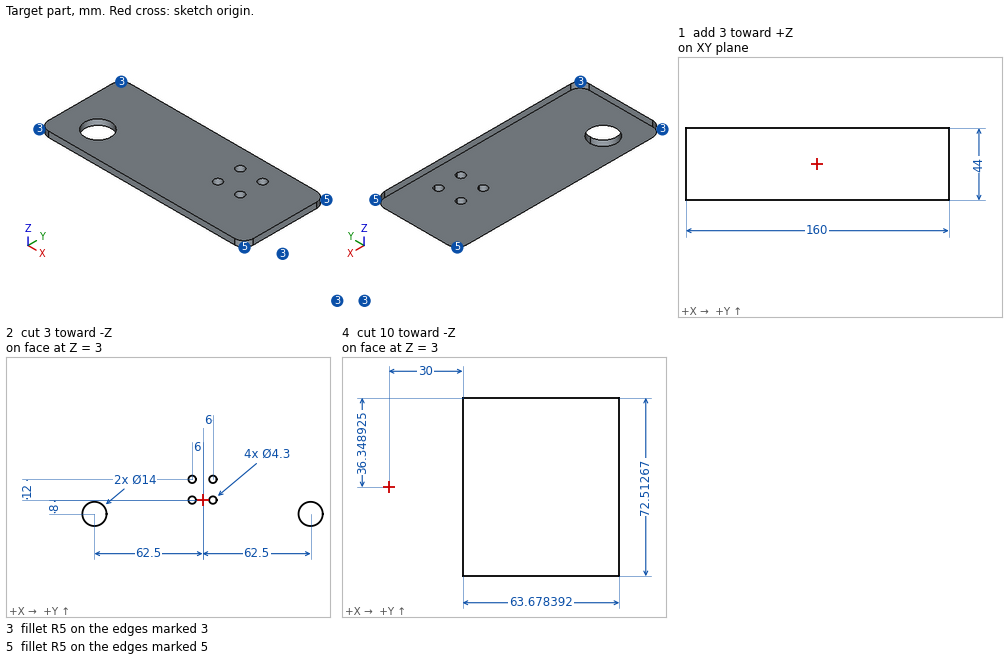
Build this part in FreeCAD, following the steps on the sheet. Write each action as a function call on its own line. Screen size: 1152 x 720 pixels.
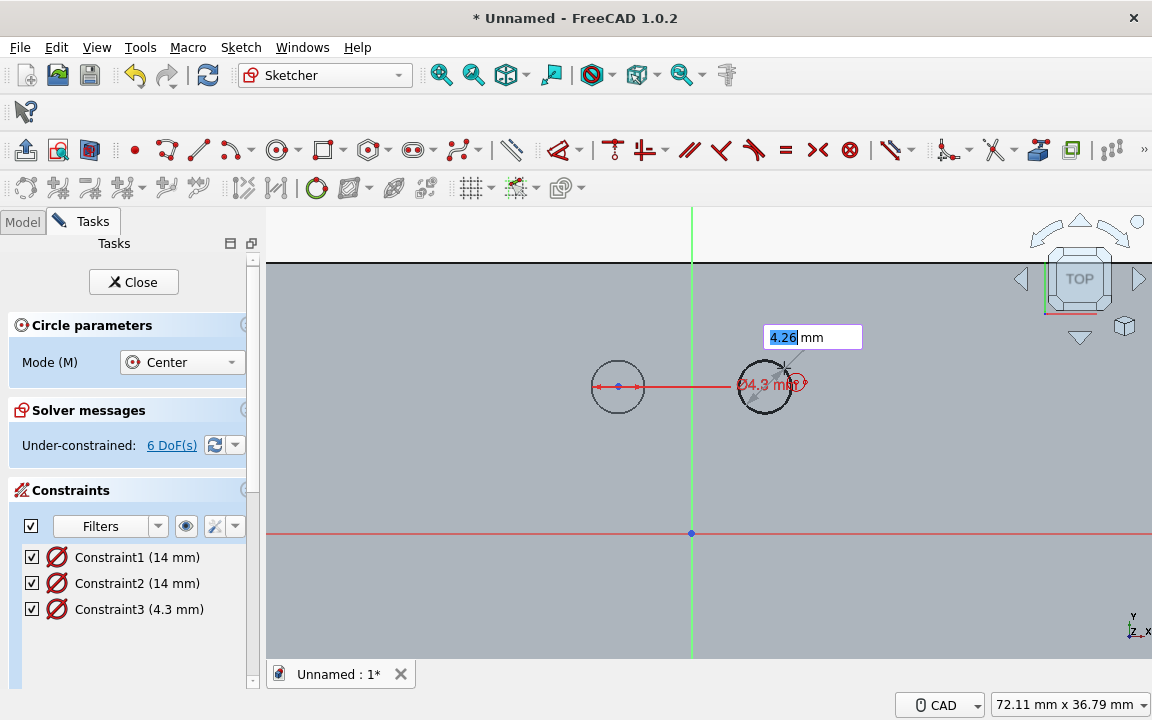
text(4.3)
key(Return)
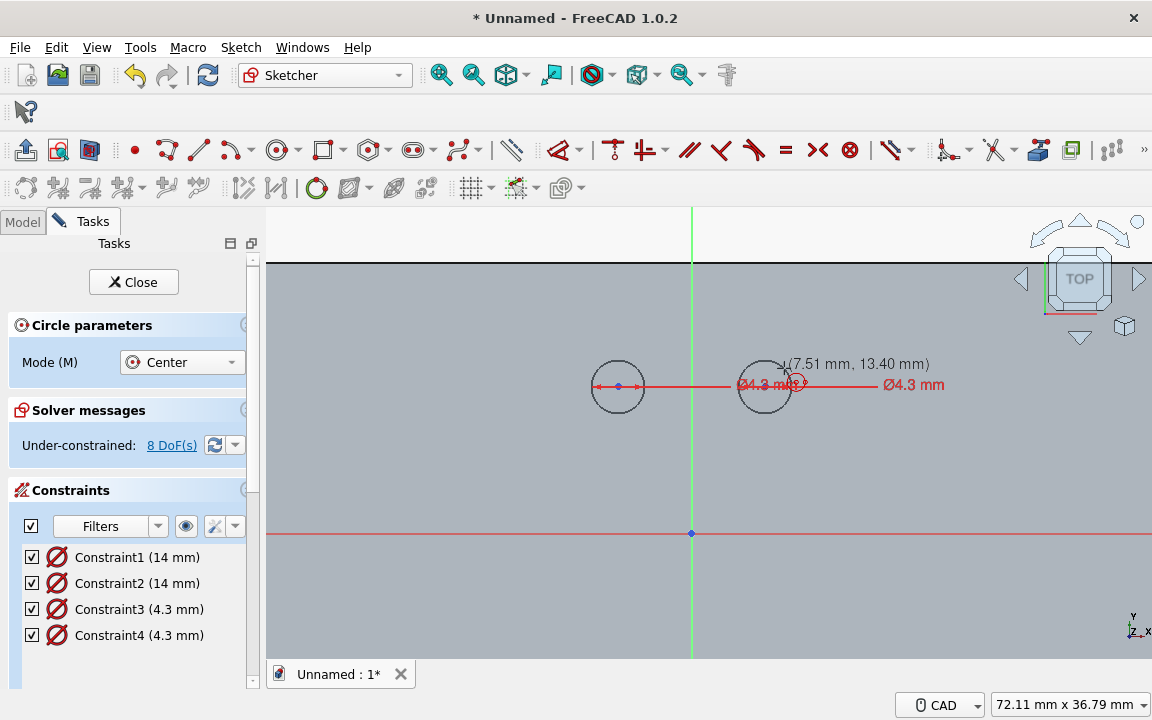
click(765, 534)
move(784, 515)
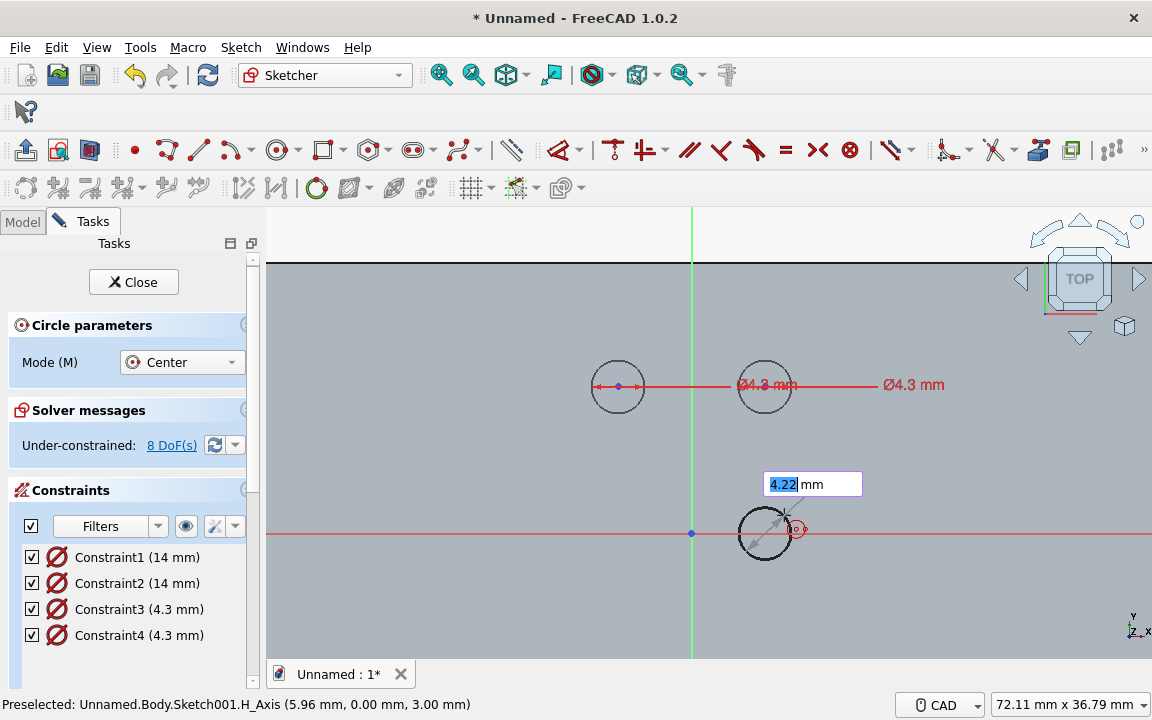
text(4.3)
key(Return)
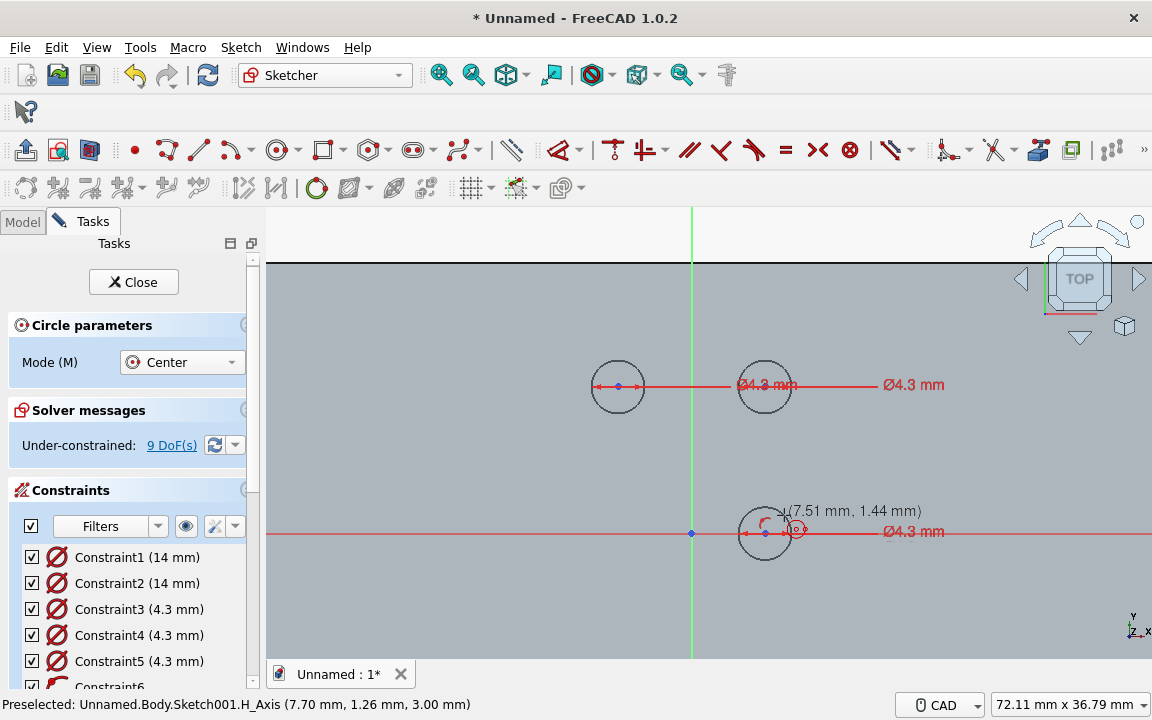
click(618, 534)
move(637, 515)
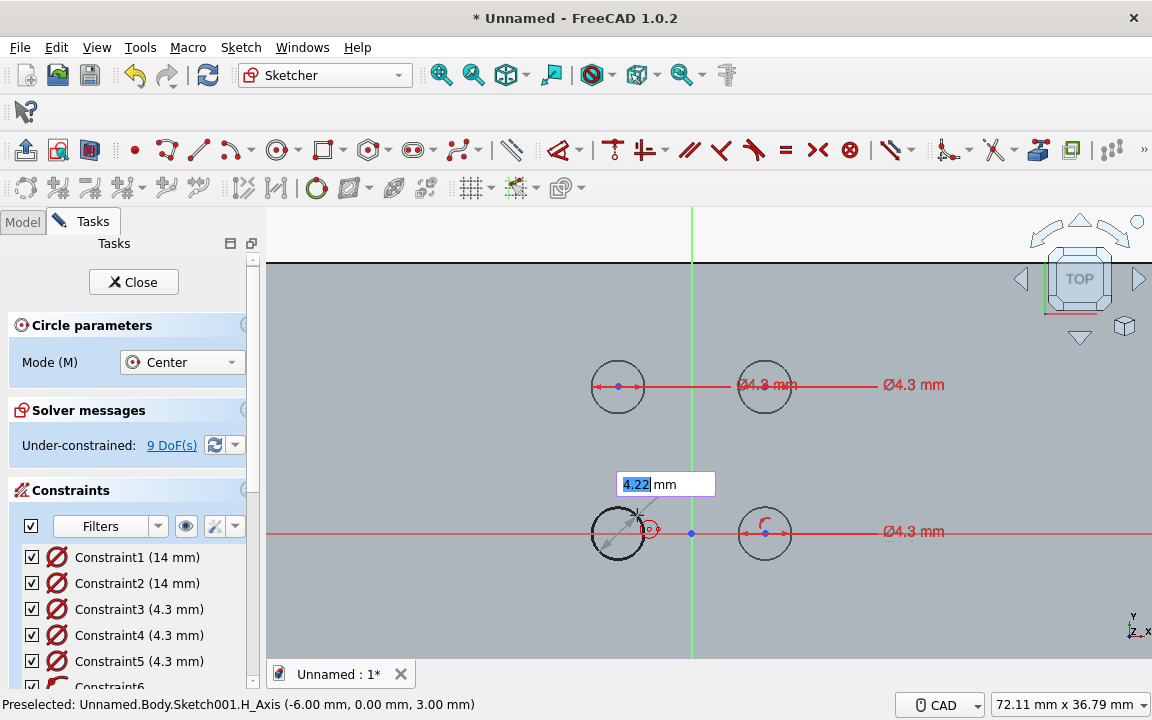
text(4.3)
key(Return)
key(Escape)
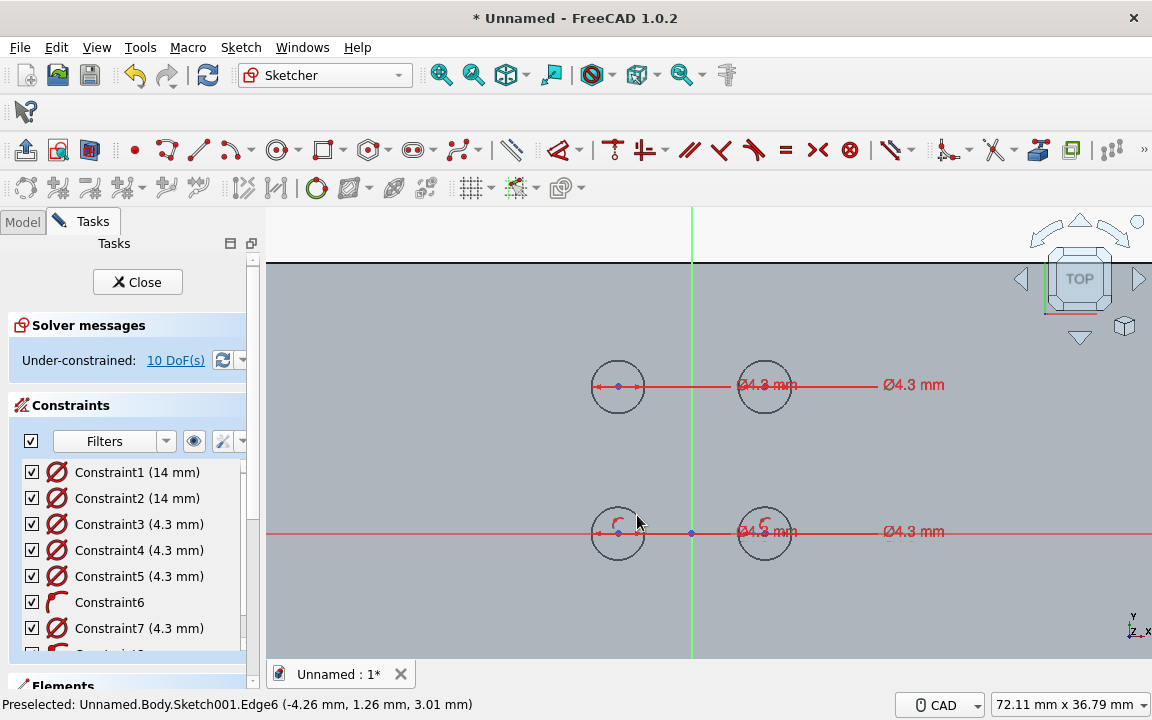
scroll(618, 387, down, 6)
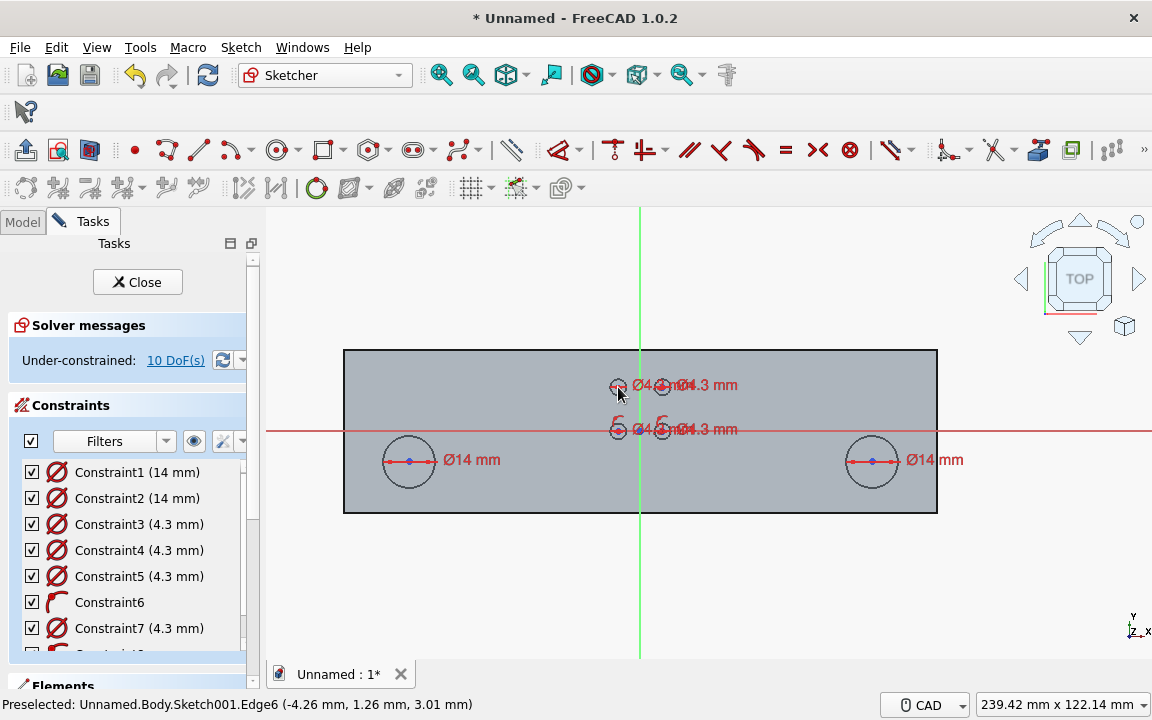
click(409, 462)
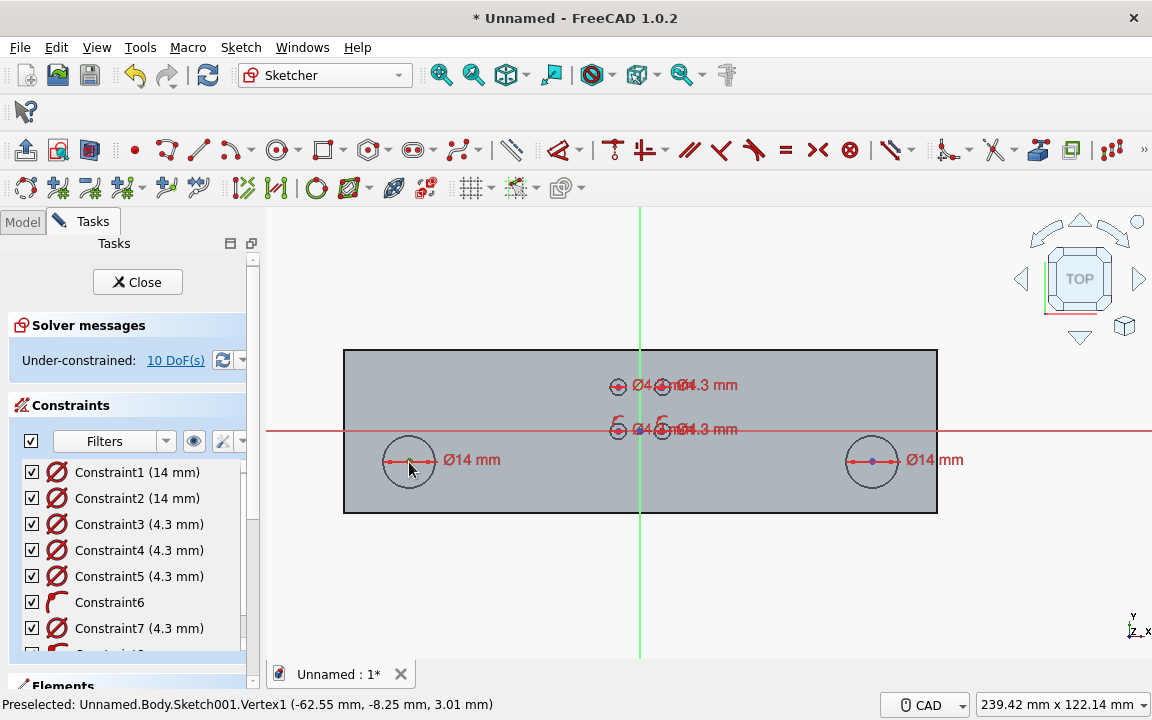
click(872, 462)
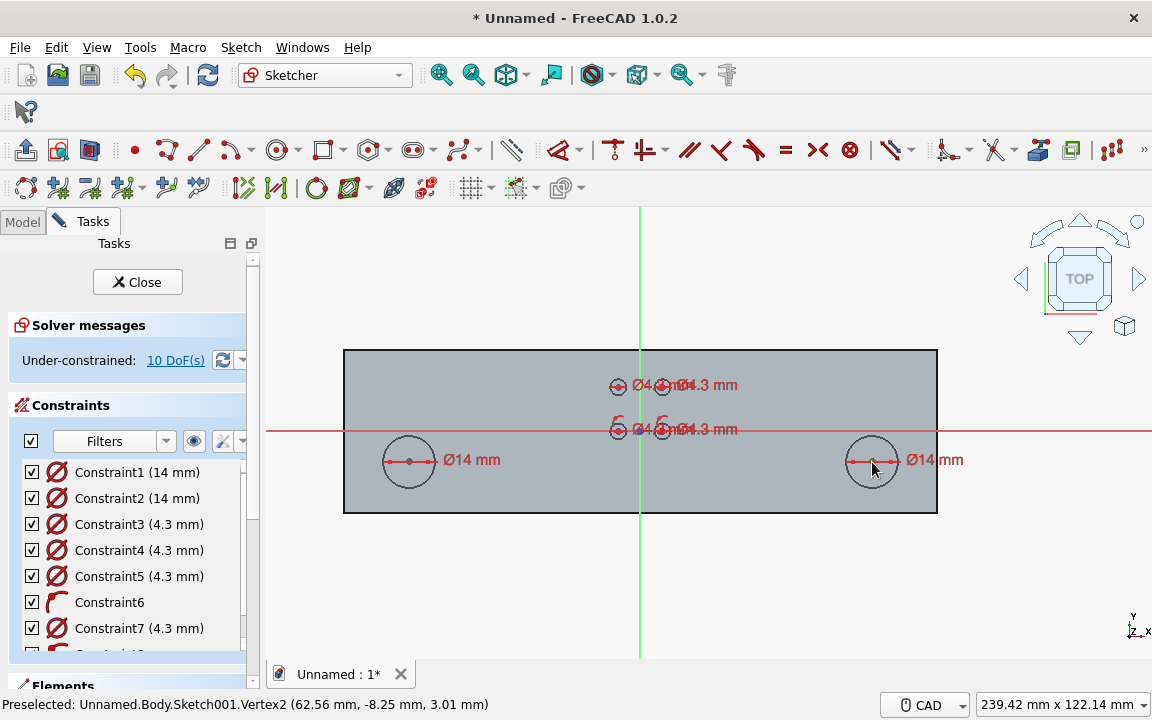
click(668, 150)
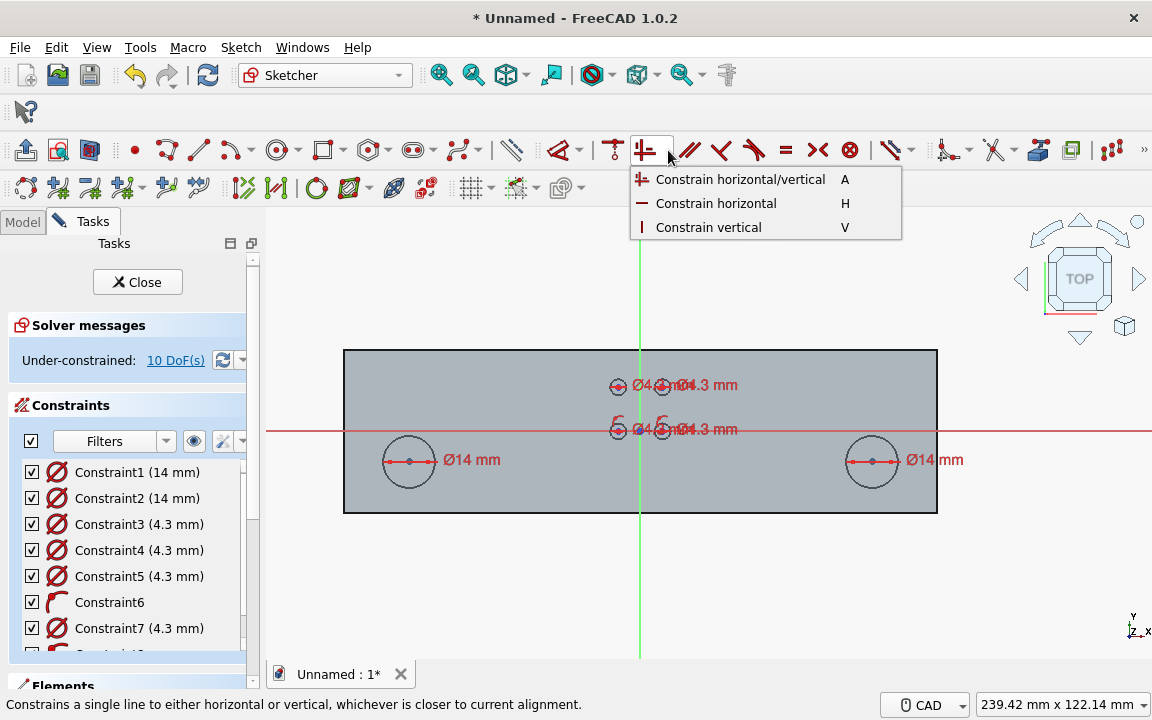
click(766, 203)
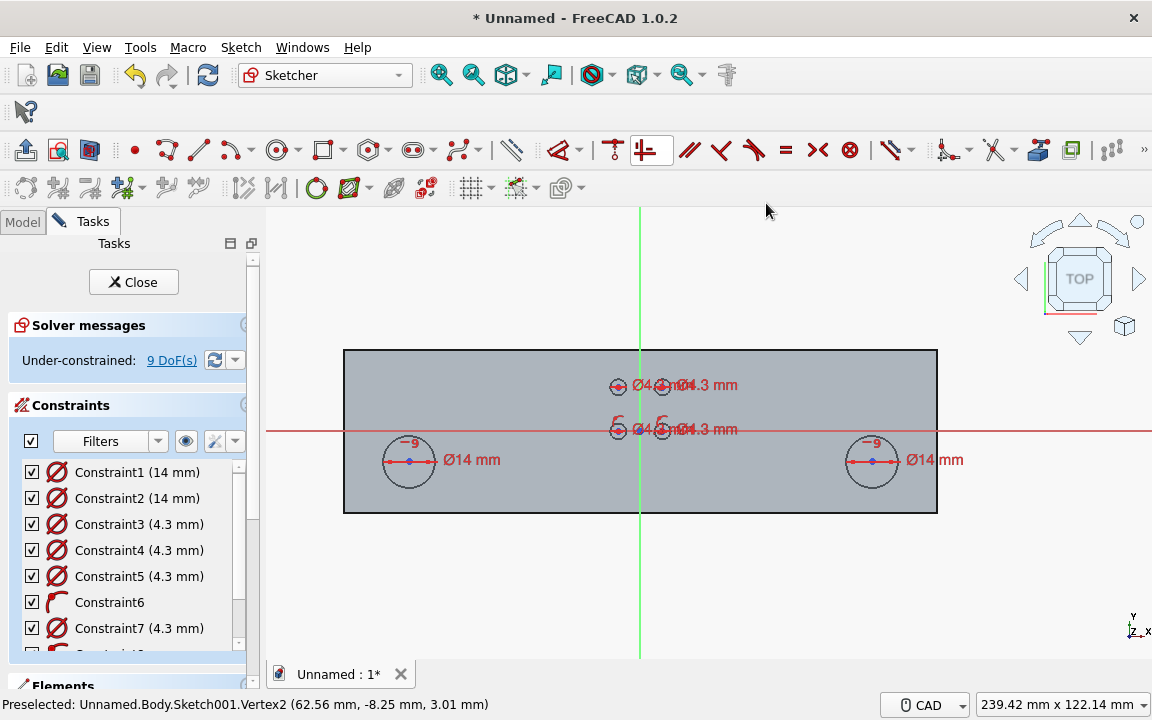
click(618, 387)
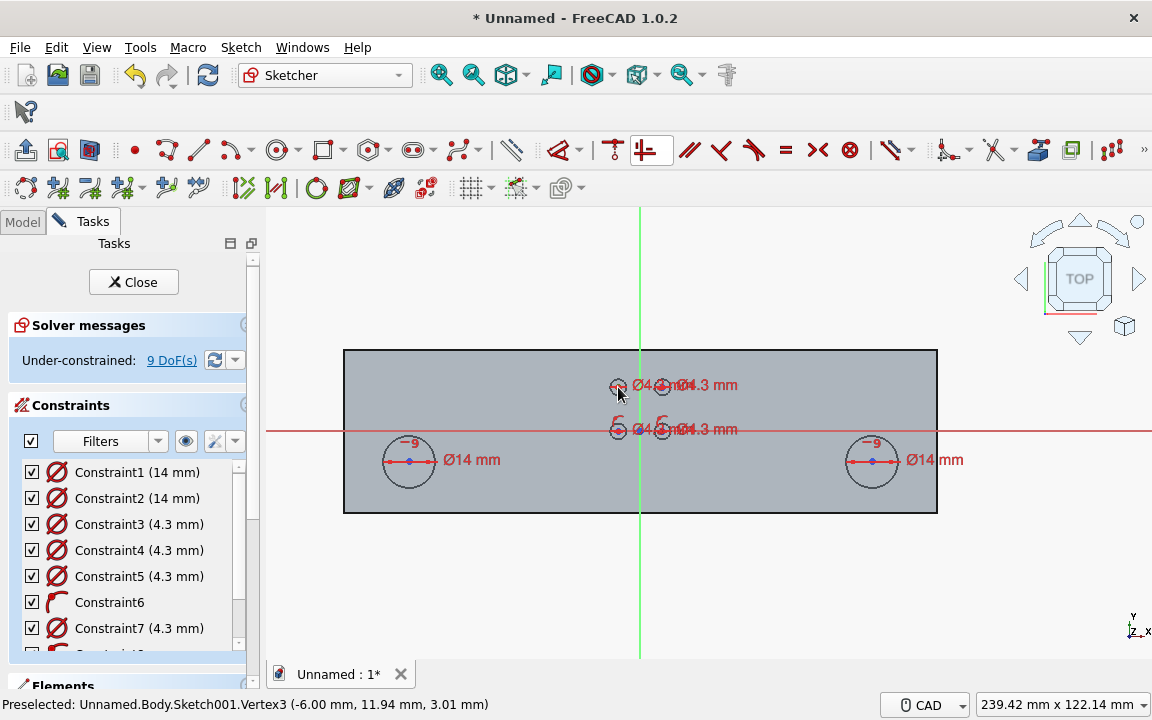
click(663, 387)